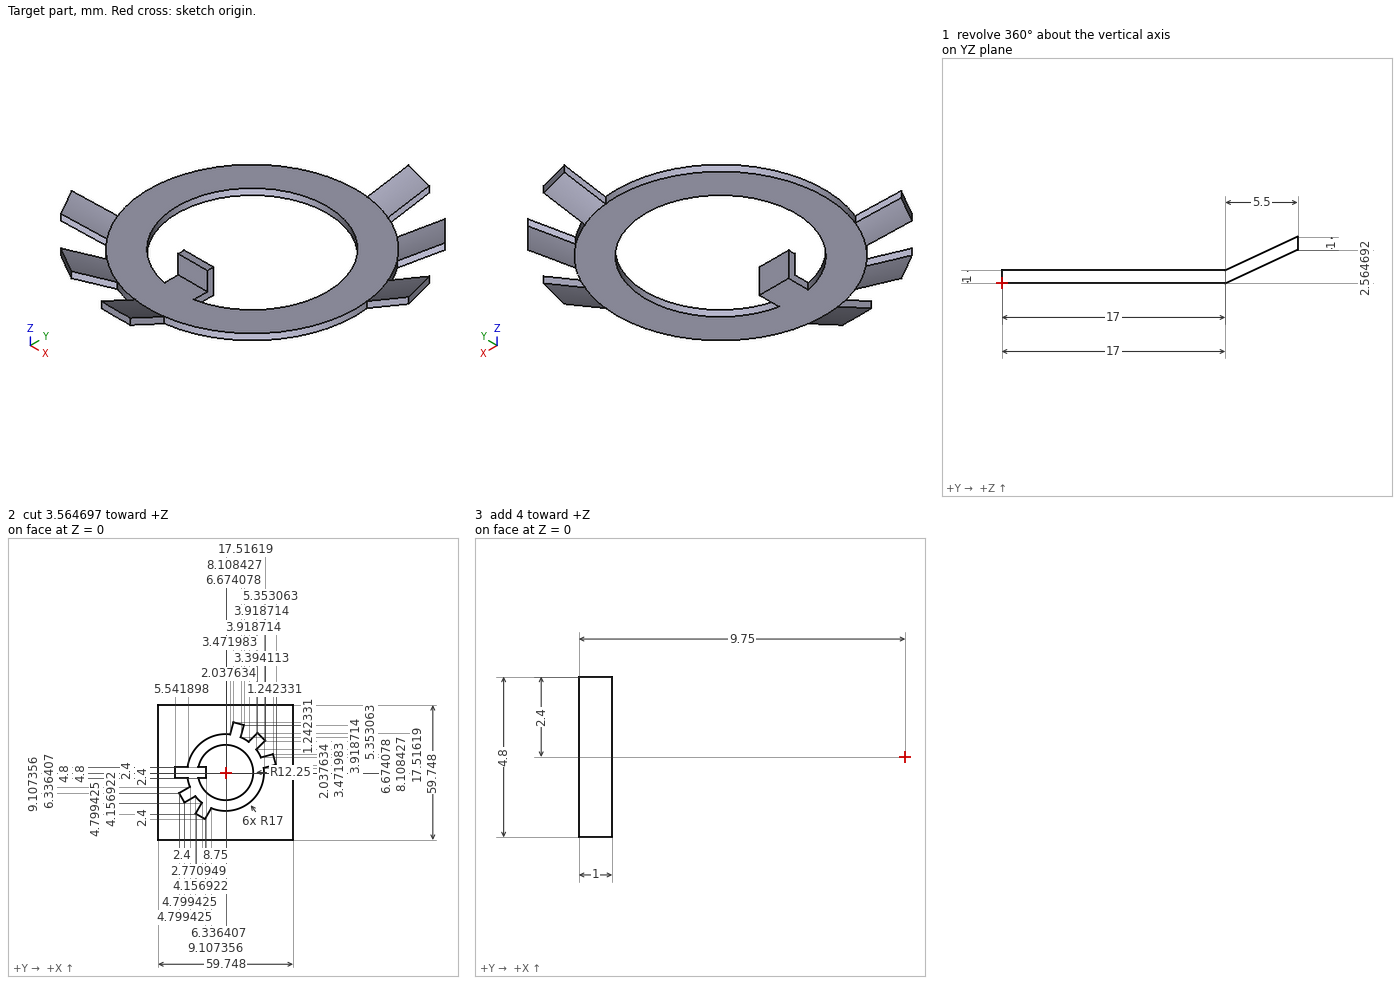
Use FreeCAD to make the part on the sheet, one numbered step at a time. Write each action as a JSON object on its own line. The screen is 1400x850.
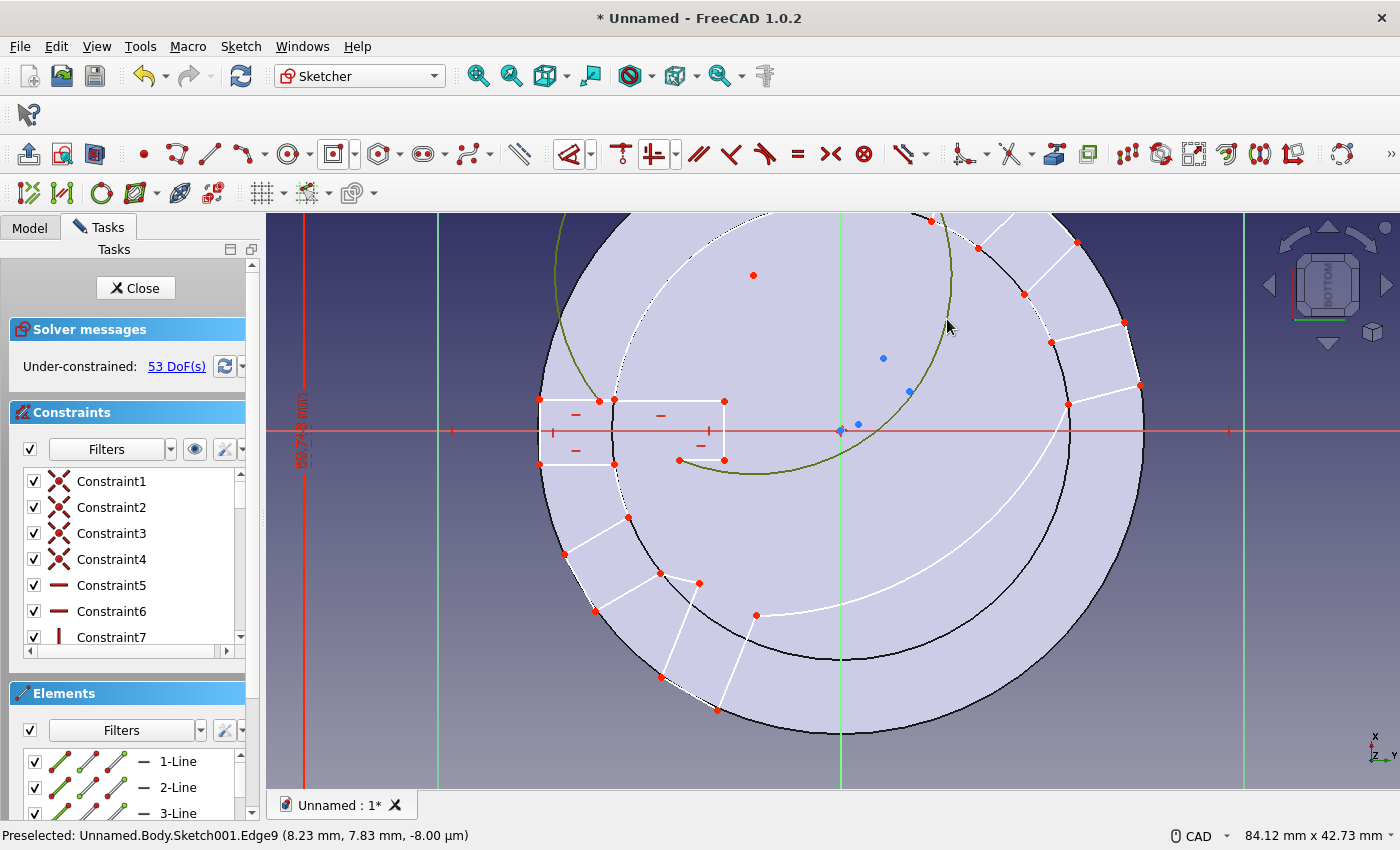
{"action": "left_click", "coordinate": [1045, 327]}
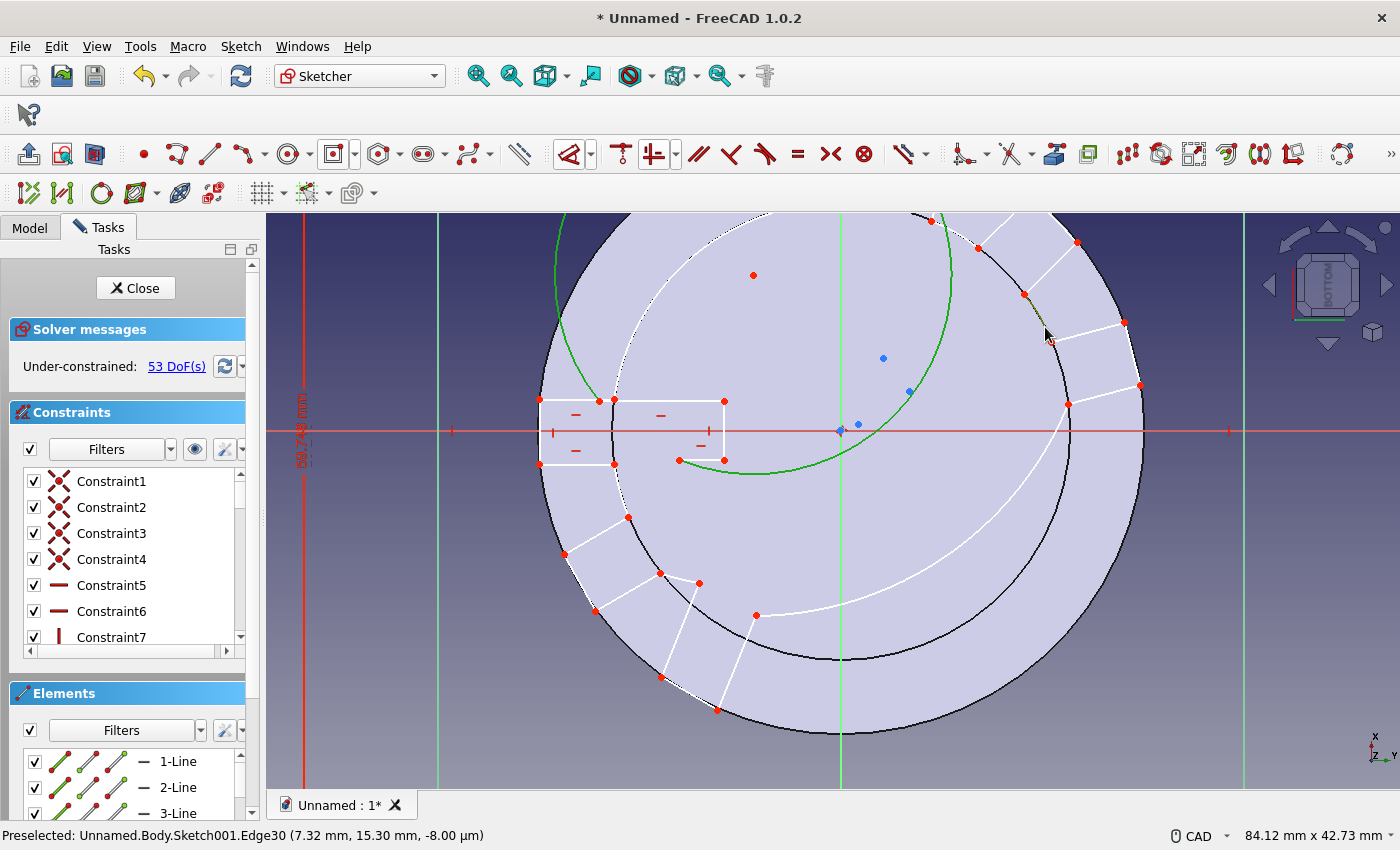
{"action": "left_click", "coordinate": [621, 154]}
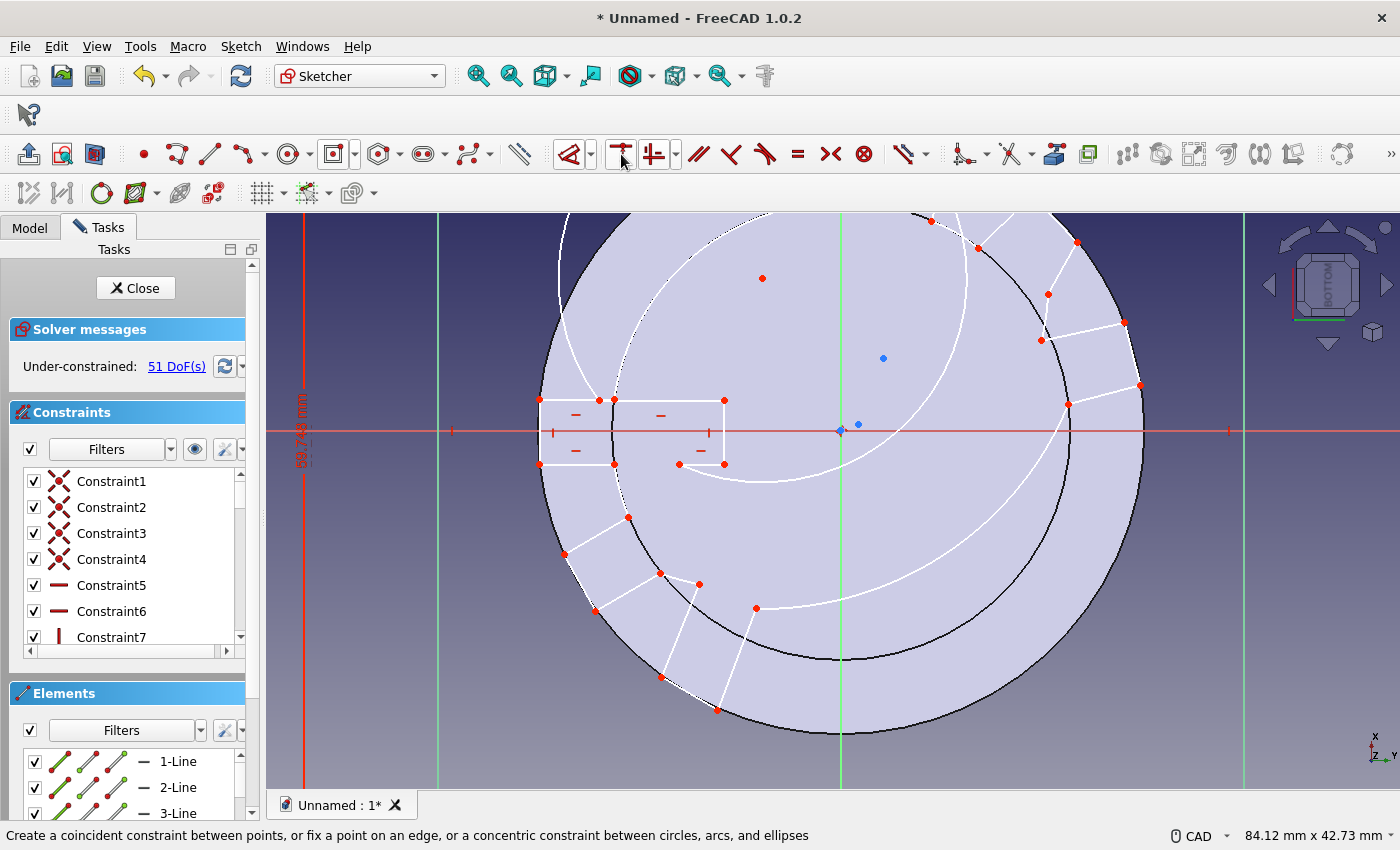
{"action": "left_click", "coordinate": [960, 330]}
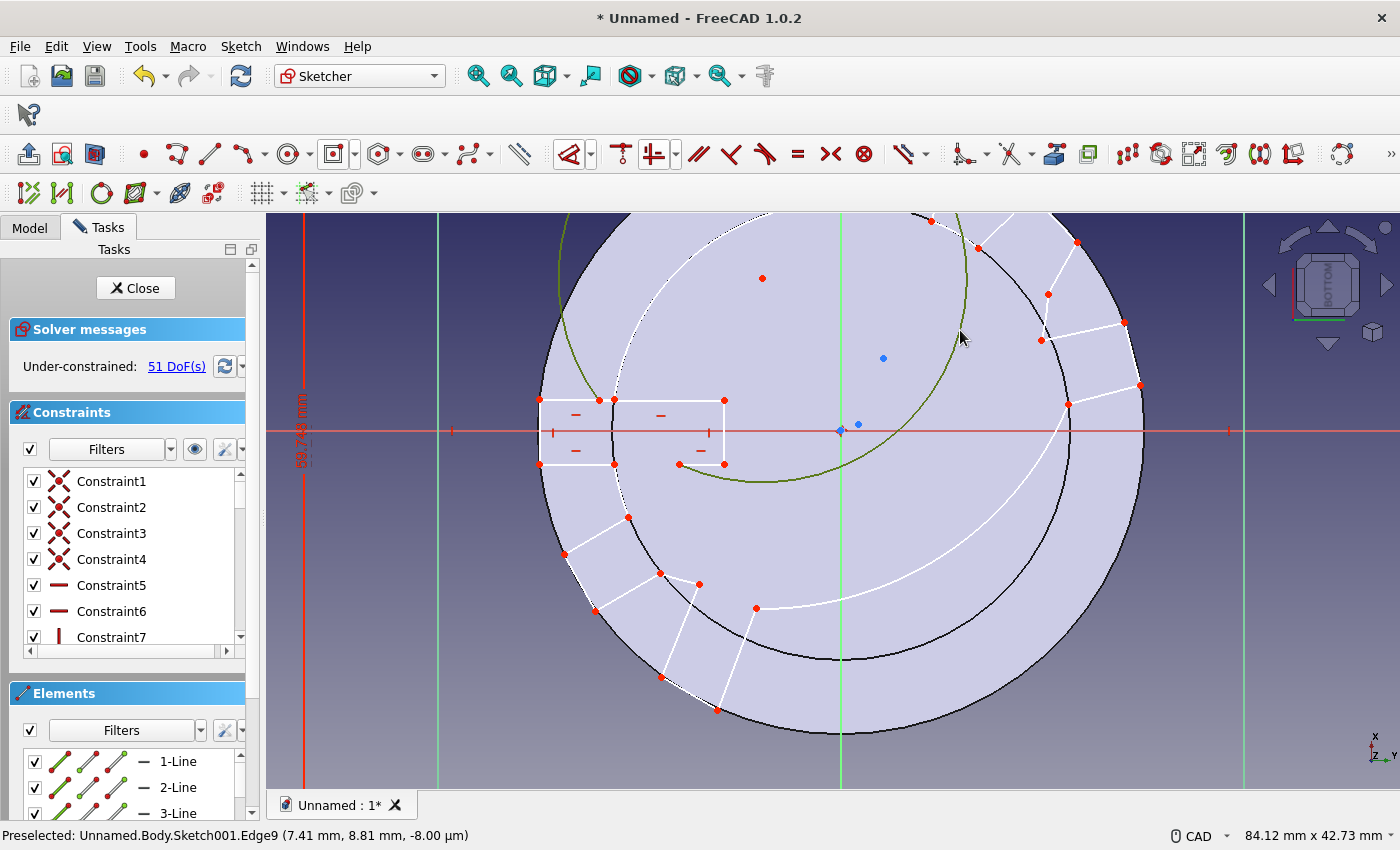
{"action": "scroll", "coordinate": [702, 558], "scroll_direction": "down", "scroll_amount": 4}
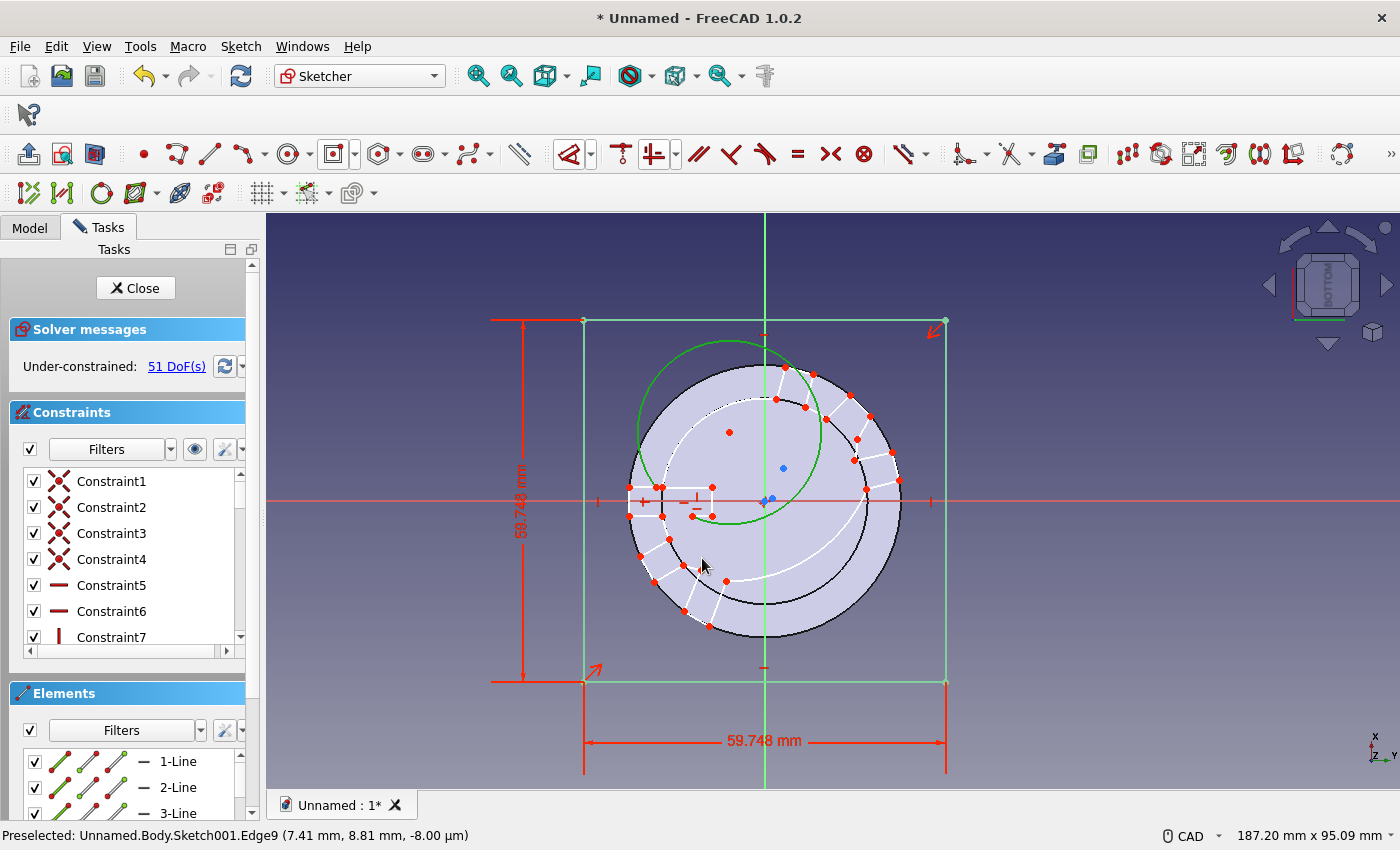
{"action": "scroll", "coordinate": [812, 410], "scroll_direction": "up", "scroll_amount": 5}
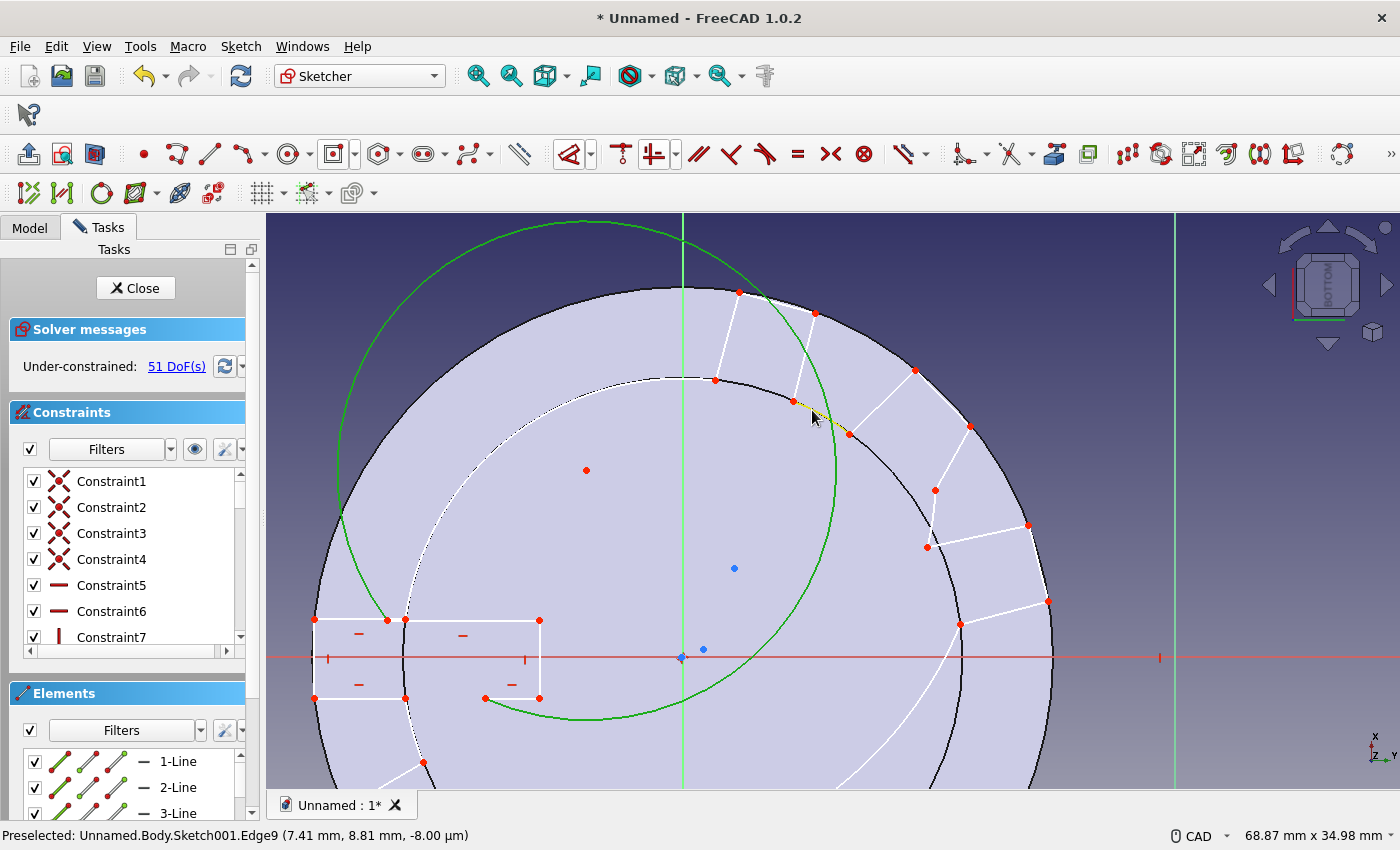
{"action": "left_click", "coordinate": [811, 409]}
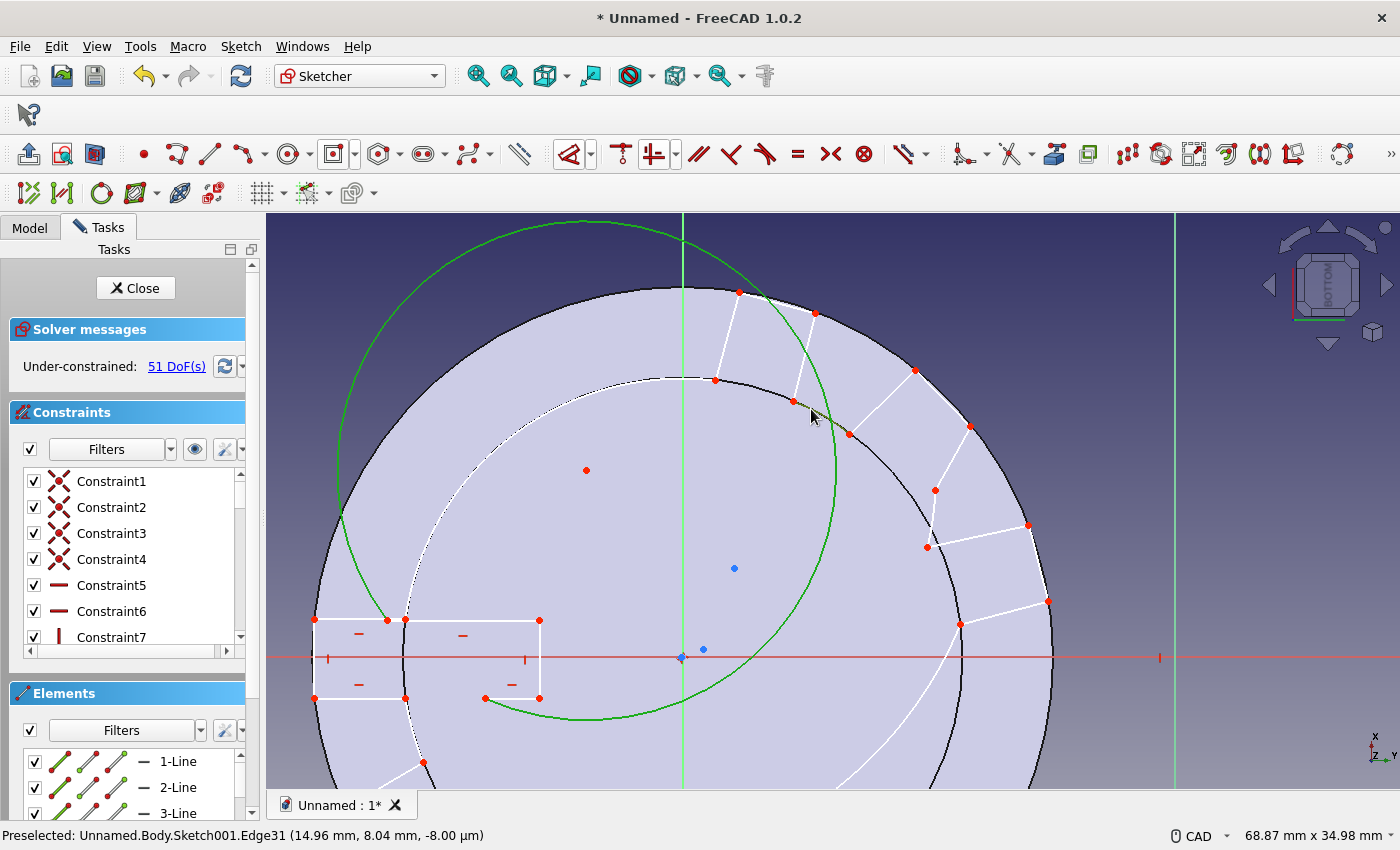
{"action": "left_click", "coordinate": [621, 154]}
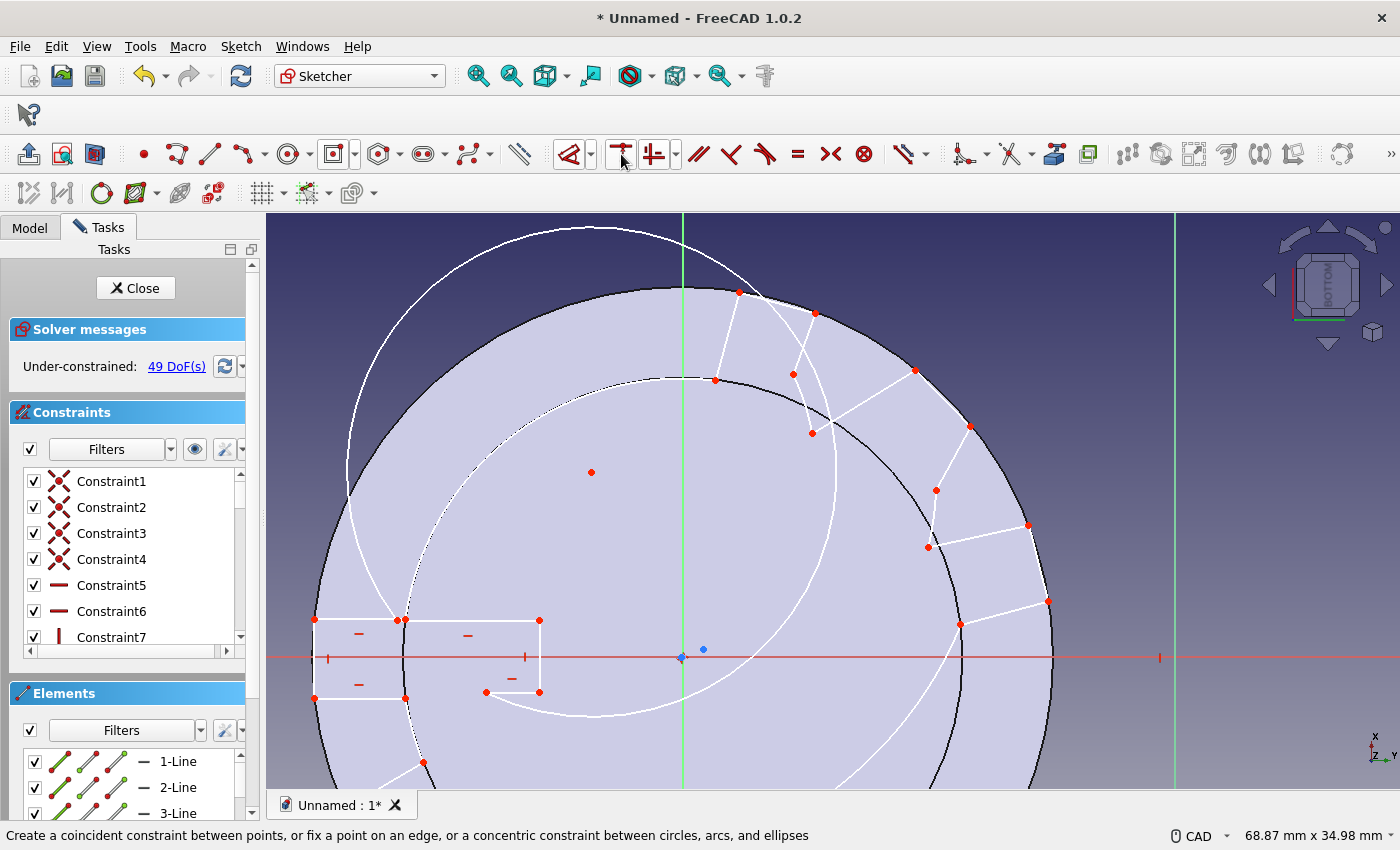
{"action": "left_click", "coordinate": [828, 538]}